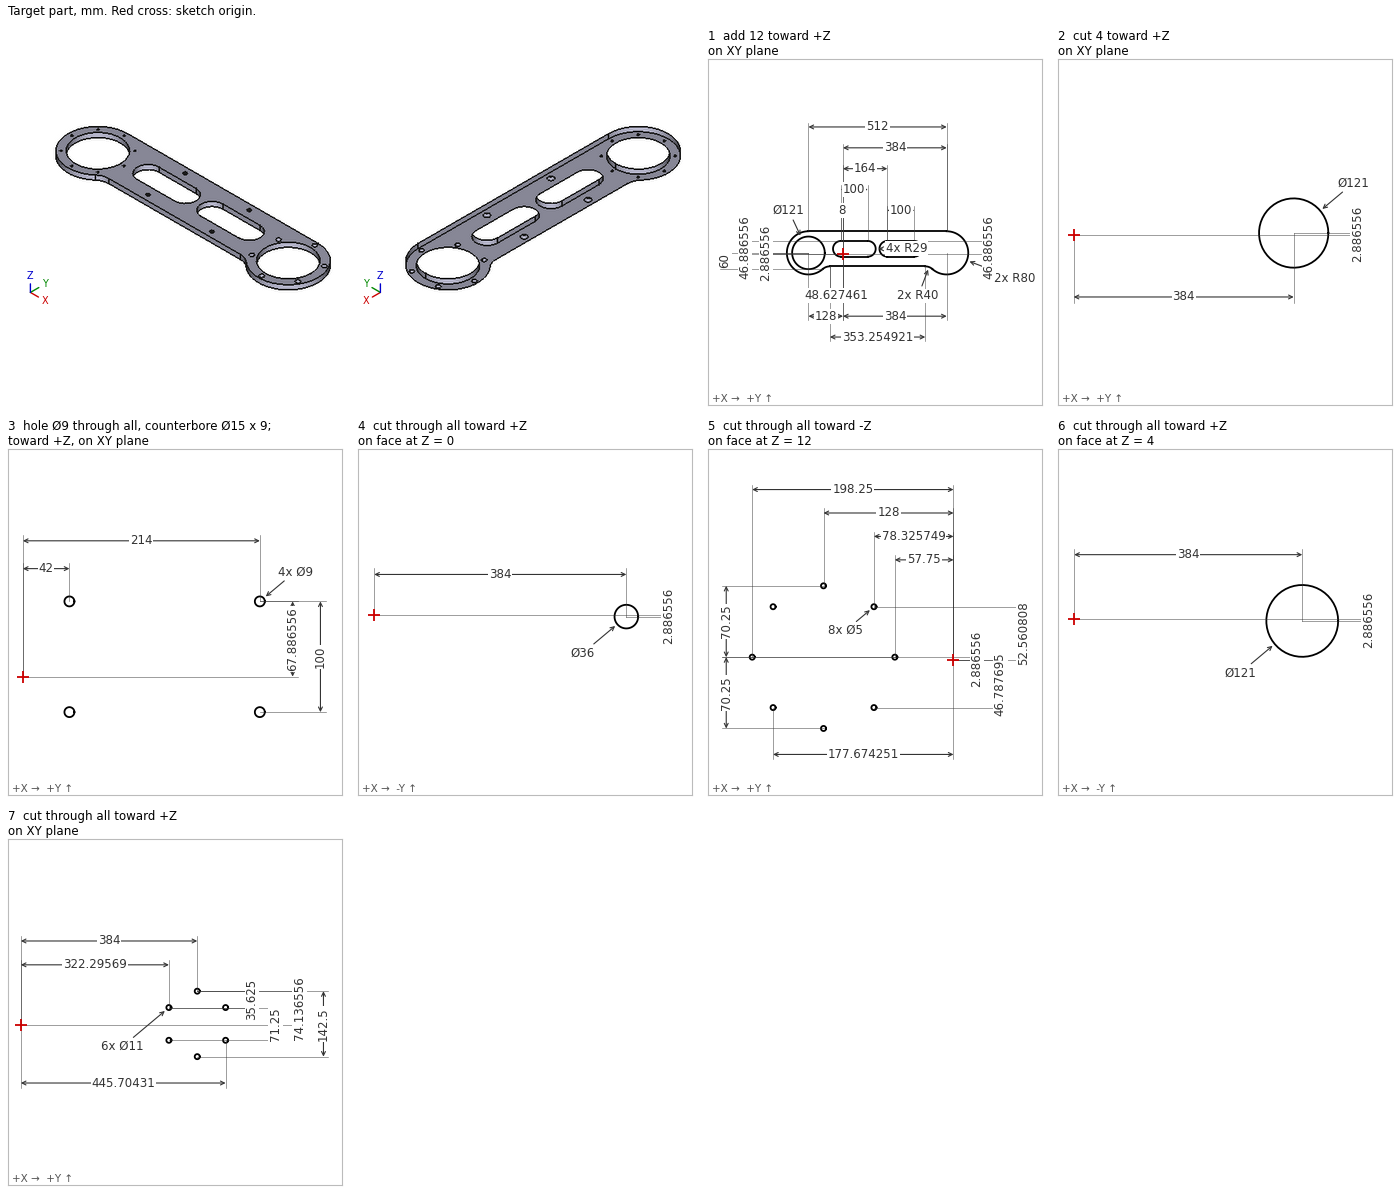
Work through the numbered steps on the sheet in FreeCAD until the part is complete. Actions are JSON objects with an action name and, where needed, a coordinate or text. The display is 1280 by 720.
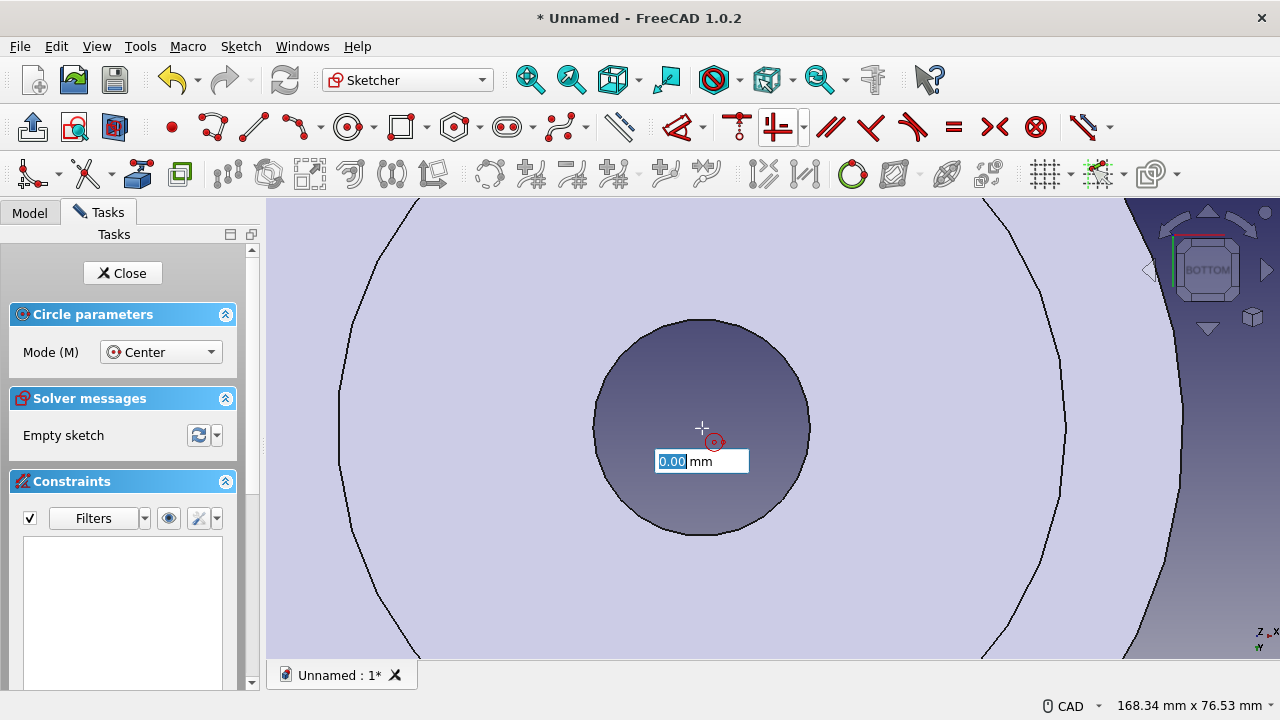
{"action": "scroll", "coordinate": [706, 429], "scroll_direction": "down", "scroll_amount": 5}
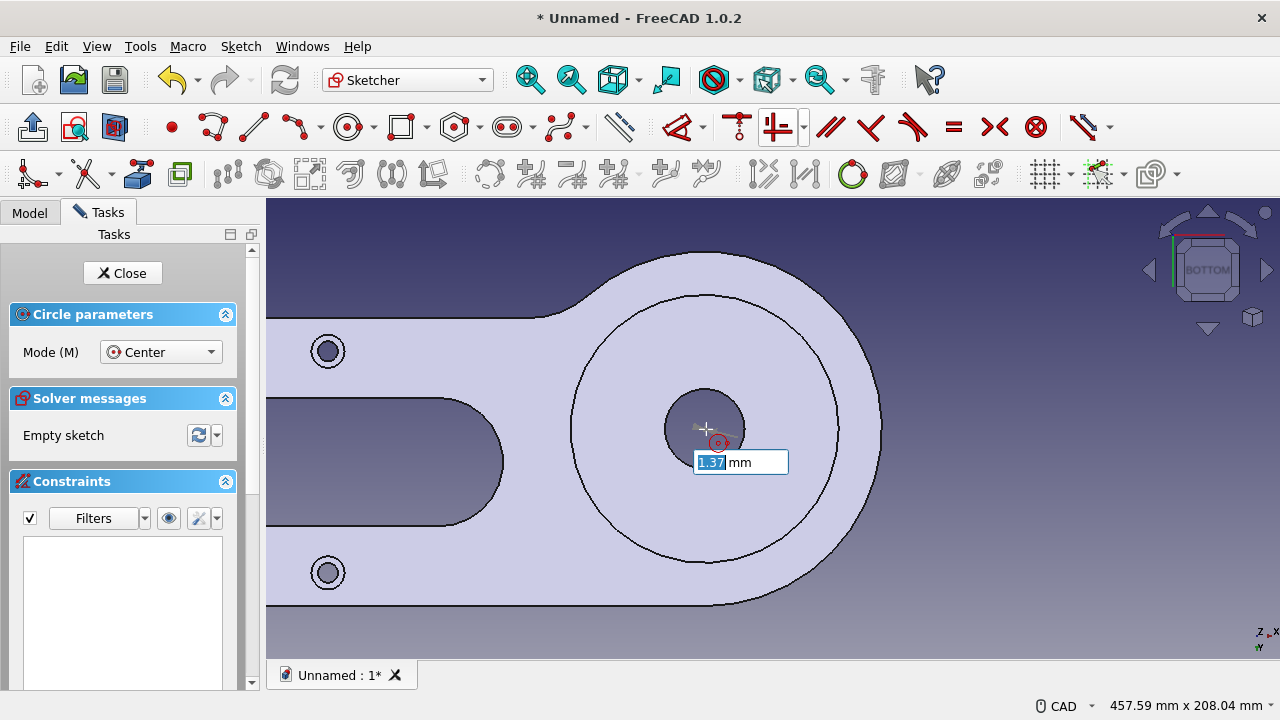
{"action": "left_click", "coordinate": [799, 334]}
{"action": "key", "text": "Escape"}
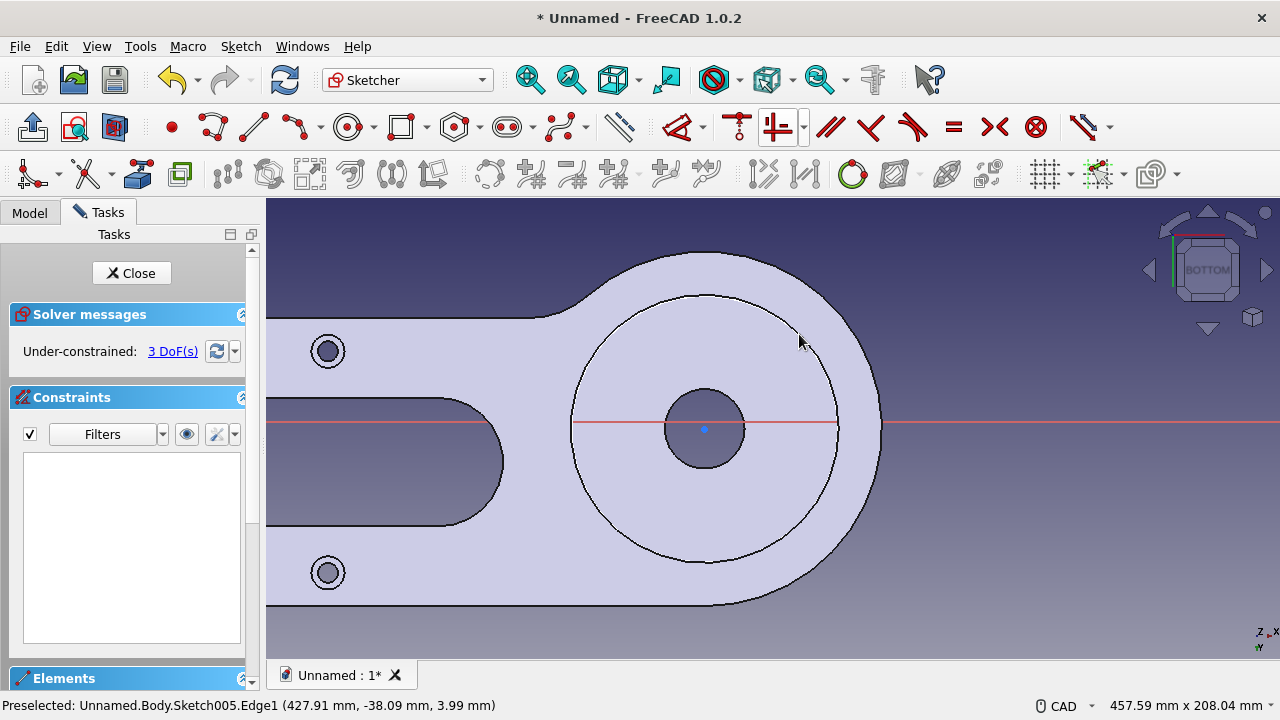
{"action": "left_click", "coordinate": [676, 128]}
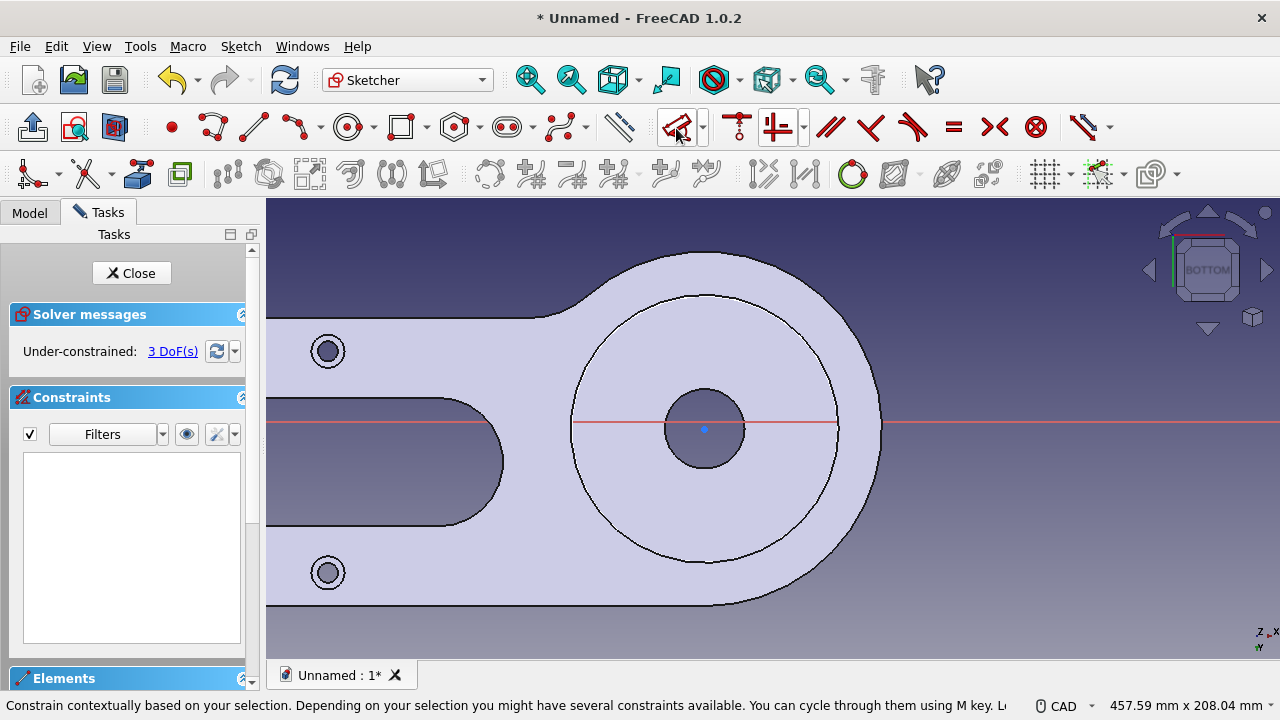
{"action": "left_click", "coordinate": [799, 335]}
{"action": "left_click", "coordinate": [822, 312]}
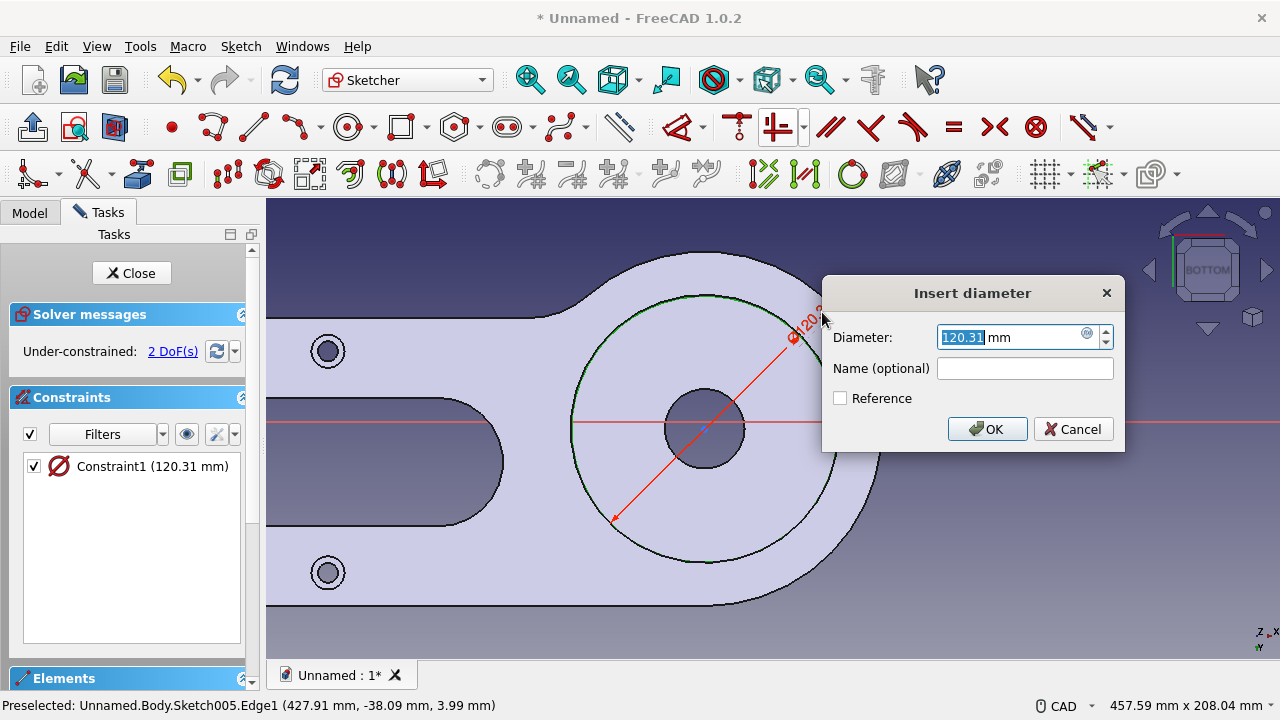
{"action": "type", "text": "121"}
{"action": "key", "text": "Return"}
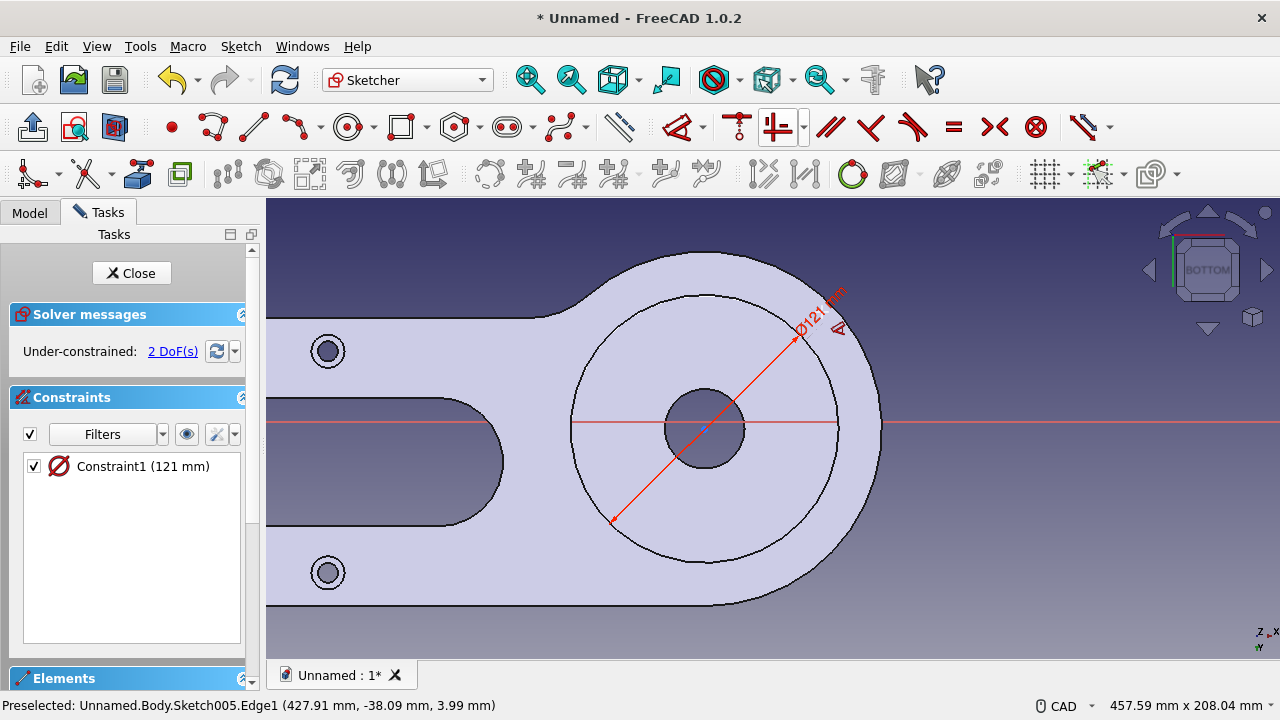
{"action": "left_click", "coordinate": [705, 429]}
{"action": "left_click", "coordinate": [499, 388]}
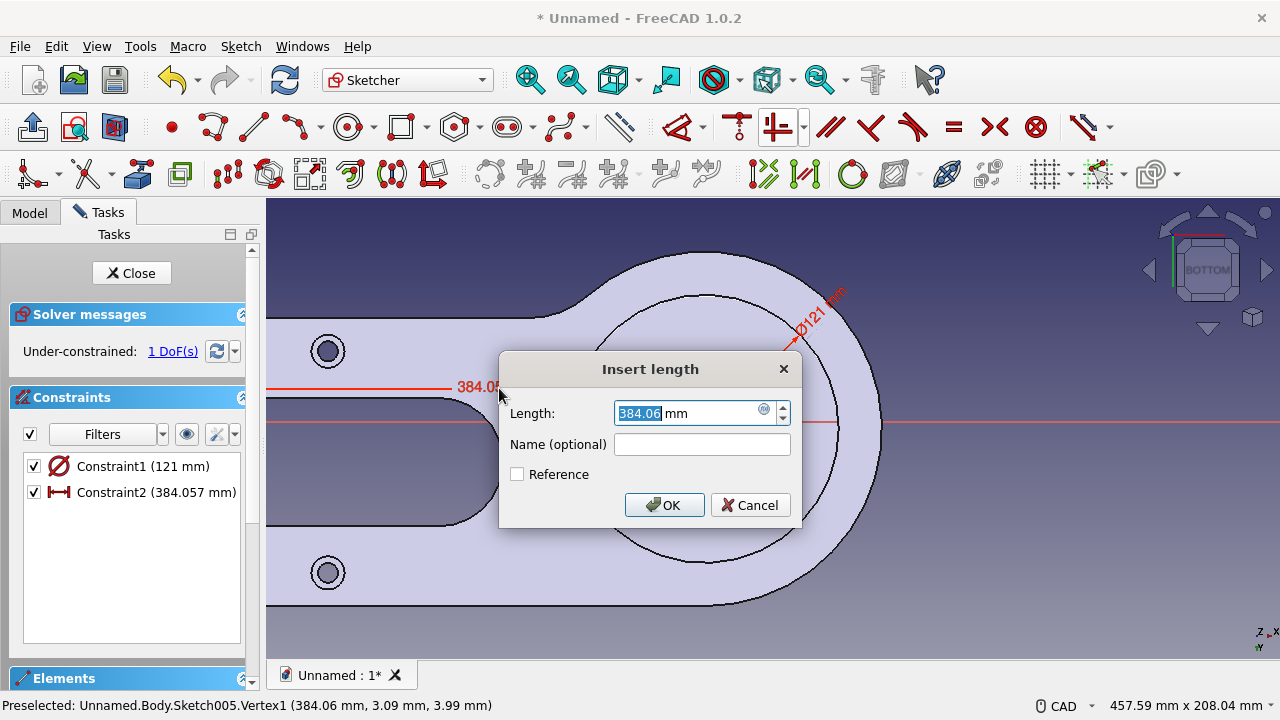
{"action": "type", "text": "384"}
{"action": "key", "text": "Return"}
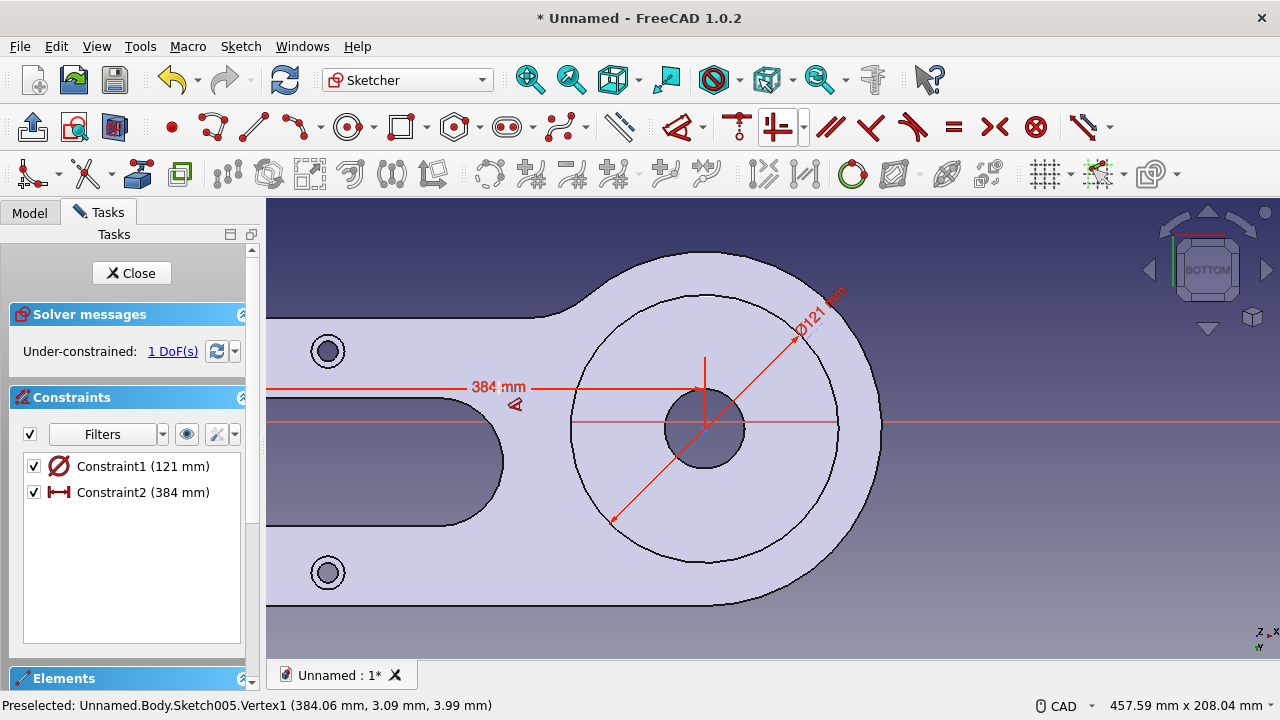
{"action": "scroll", "coordinate": [705, 429], "scroll_direction": "up", "scroll_amount": 10}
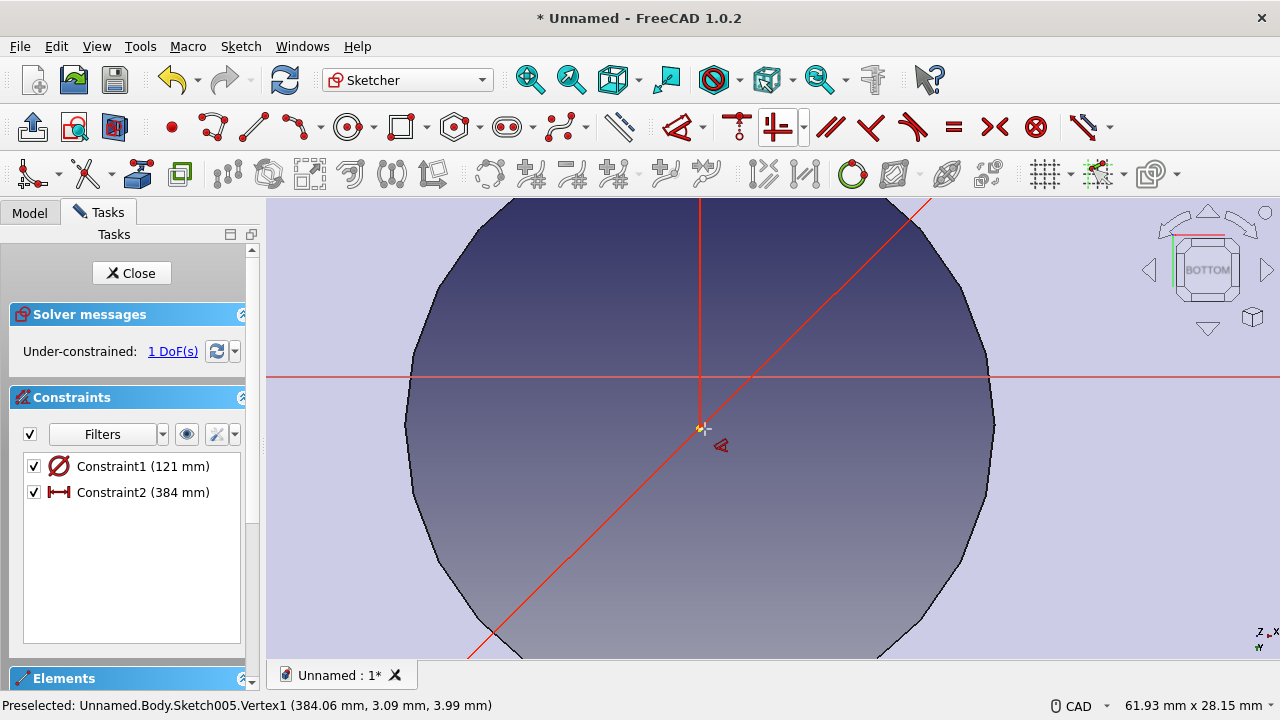
{"action": "left_click", "coordinate": [700, 428]}
{"action": "left_click", "coordinate": [734, 403]}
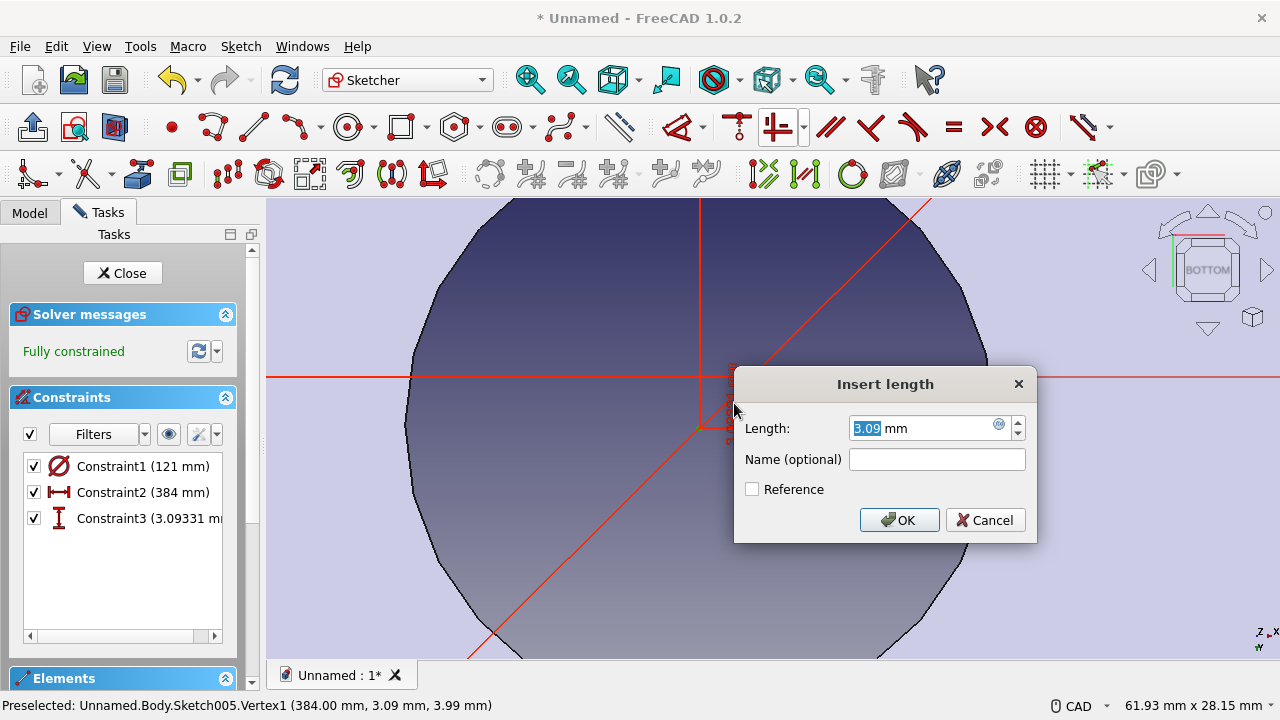
{"action": "type", "text": "2.886556"}
{"action": "key", "text": "Return"}
{"action": "key", "text": "Escape"}